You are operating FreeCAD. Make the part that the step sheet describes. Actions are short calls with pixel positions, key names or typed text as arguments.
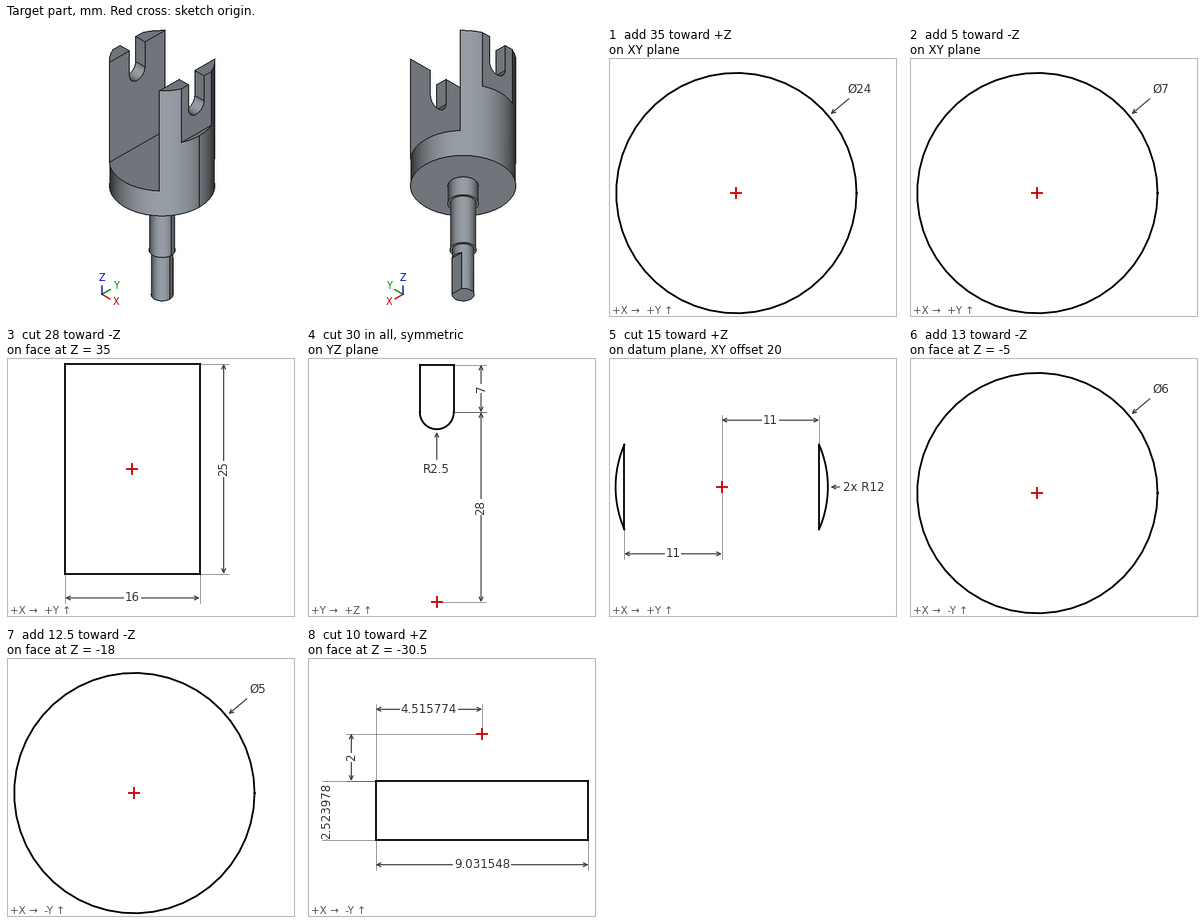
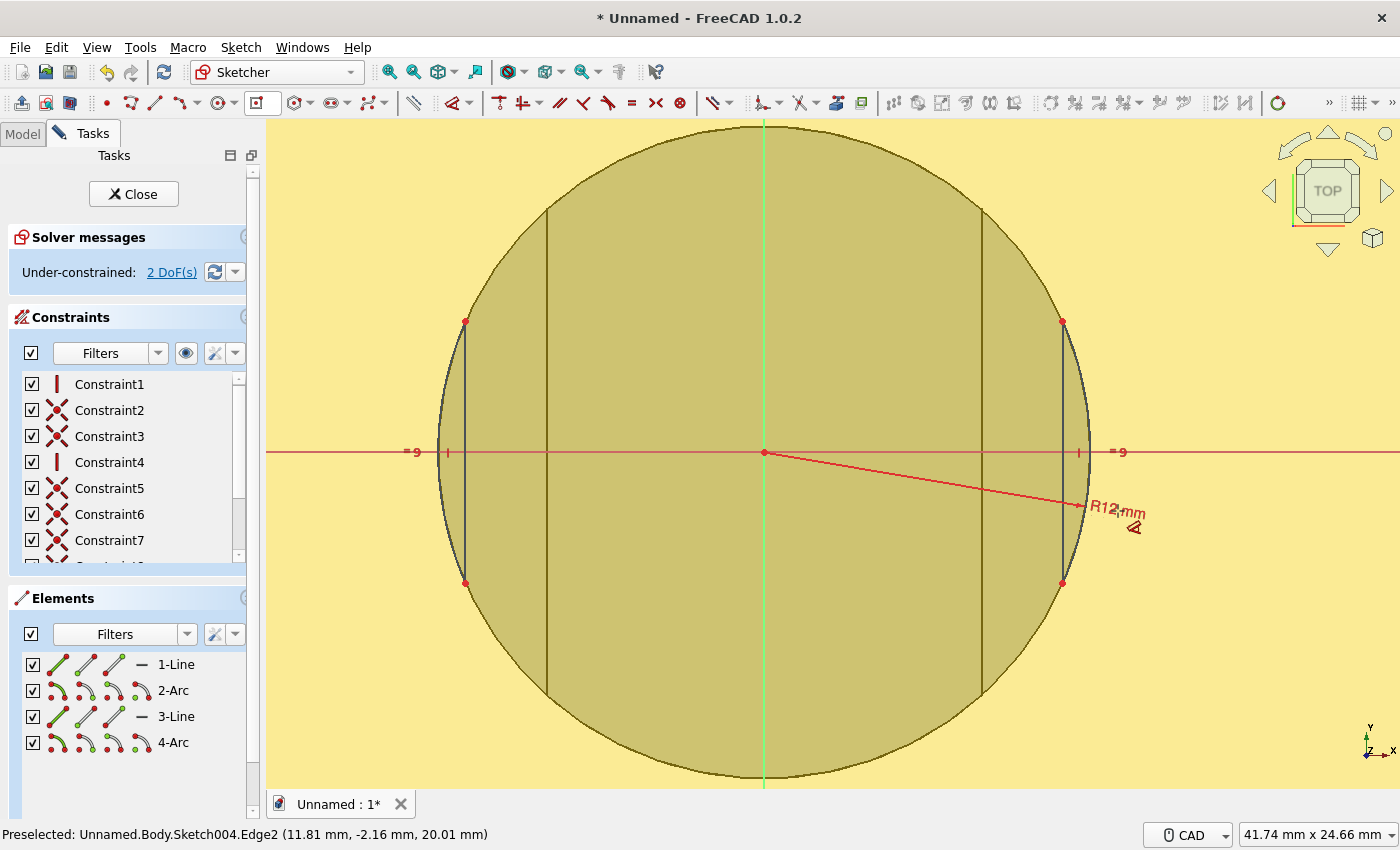
click(1063, 322)
click(914, 288)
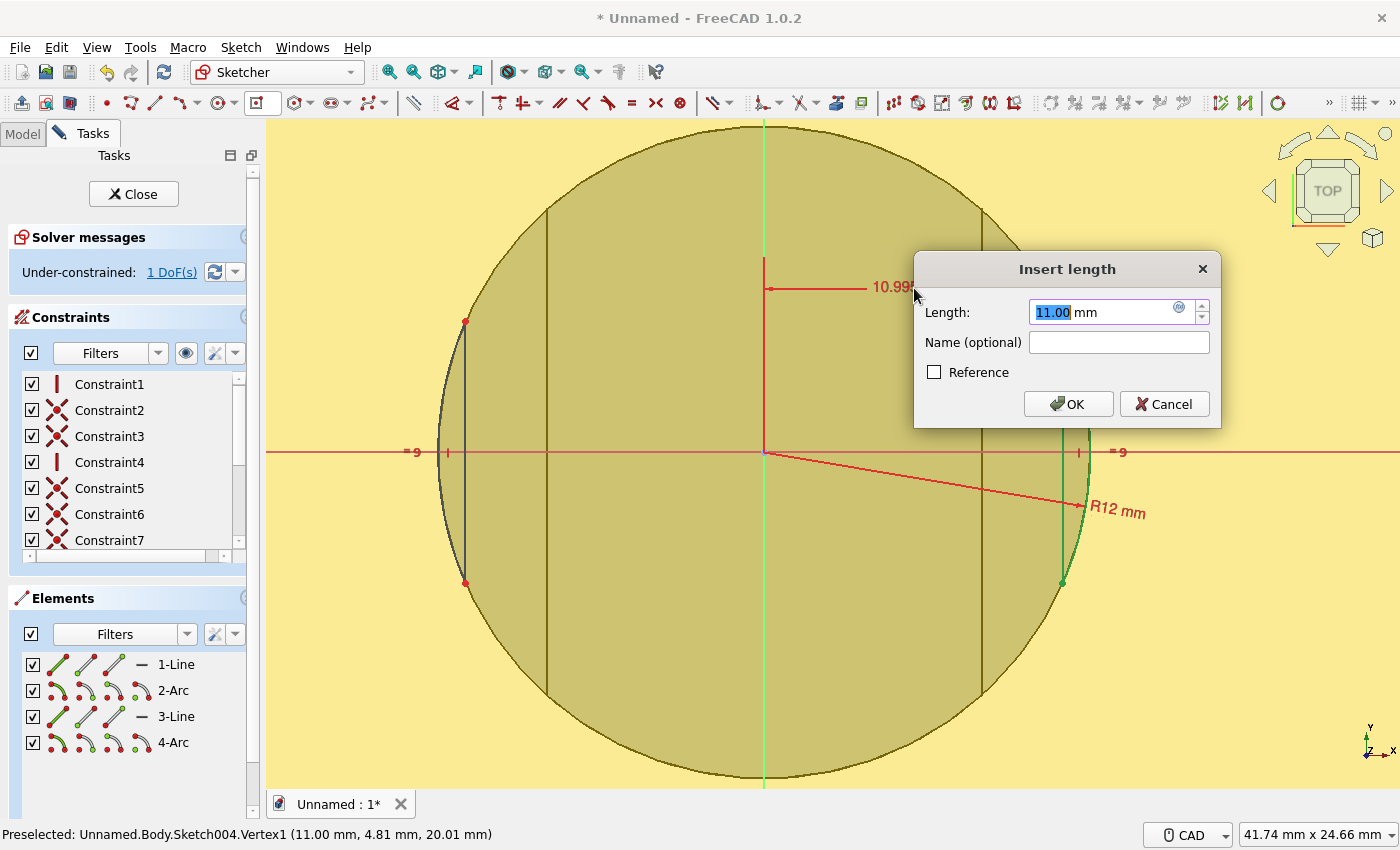
text(11)
key(Return)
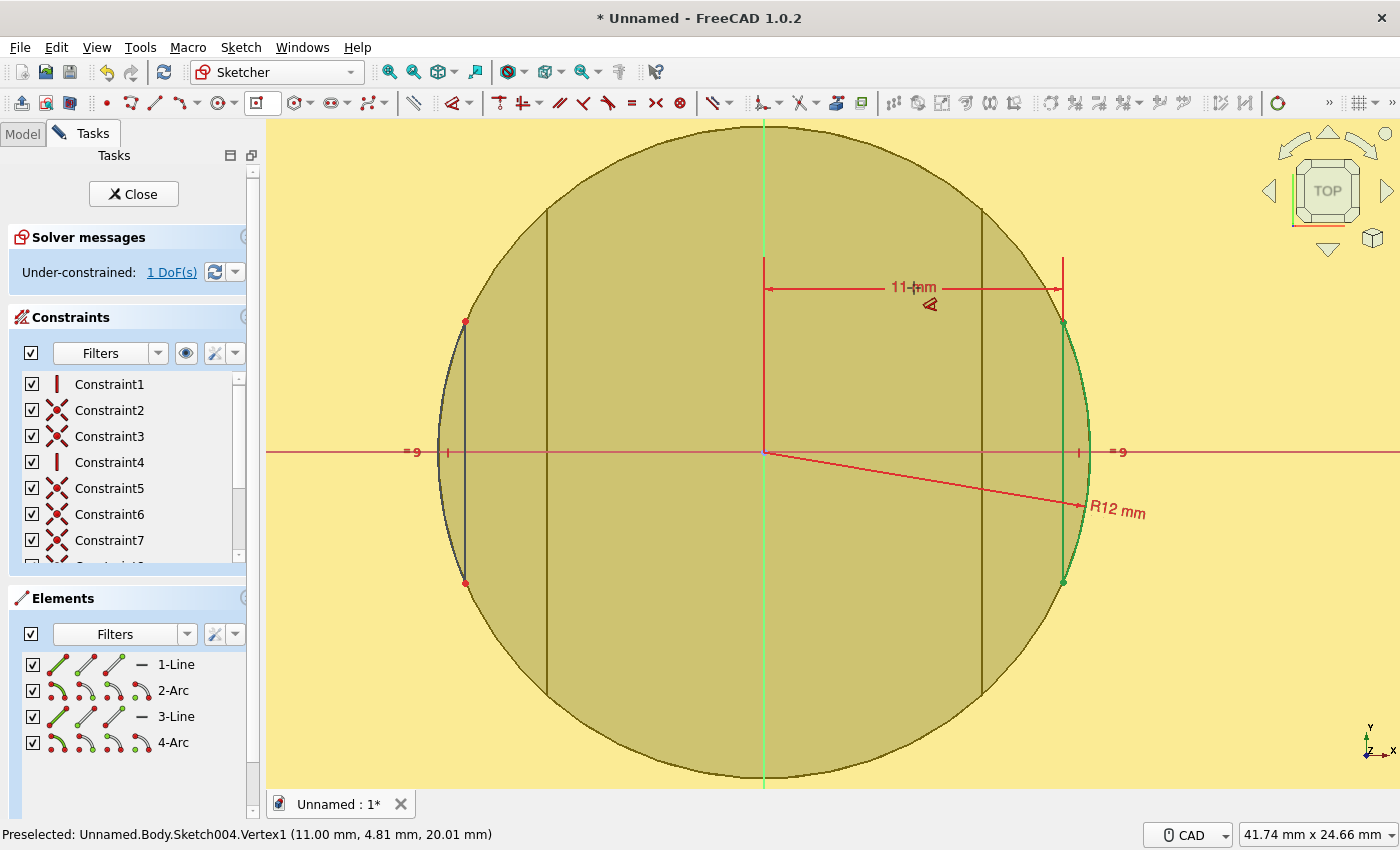
click(465, 583)
click(615, 617)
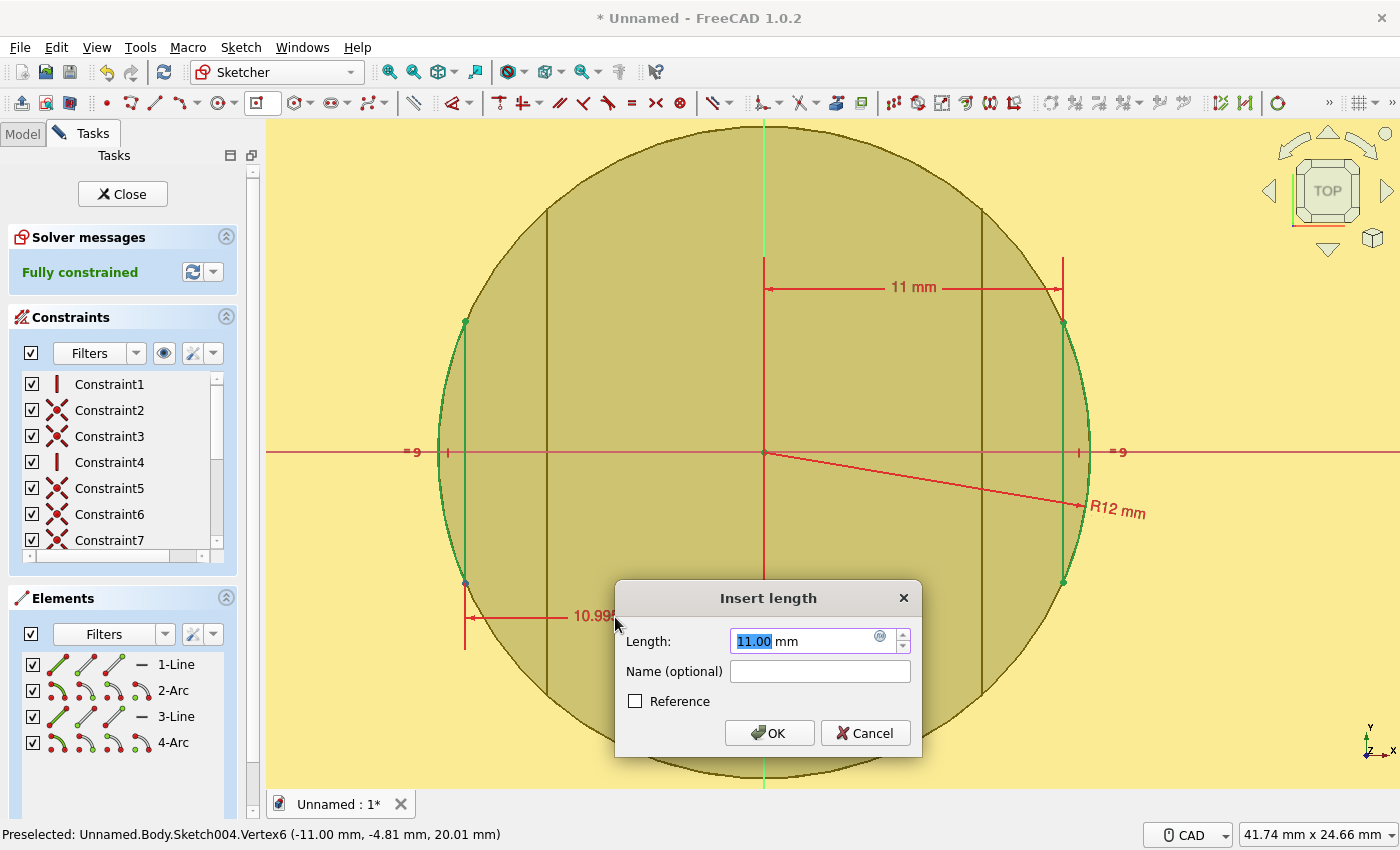
text(11)
key(Return)
key(Escape)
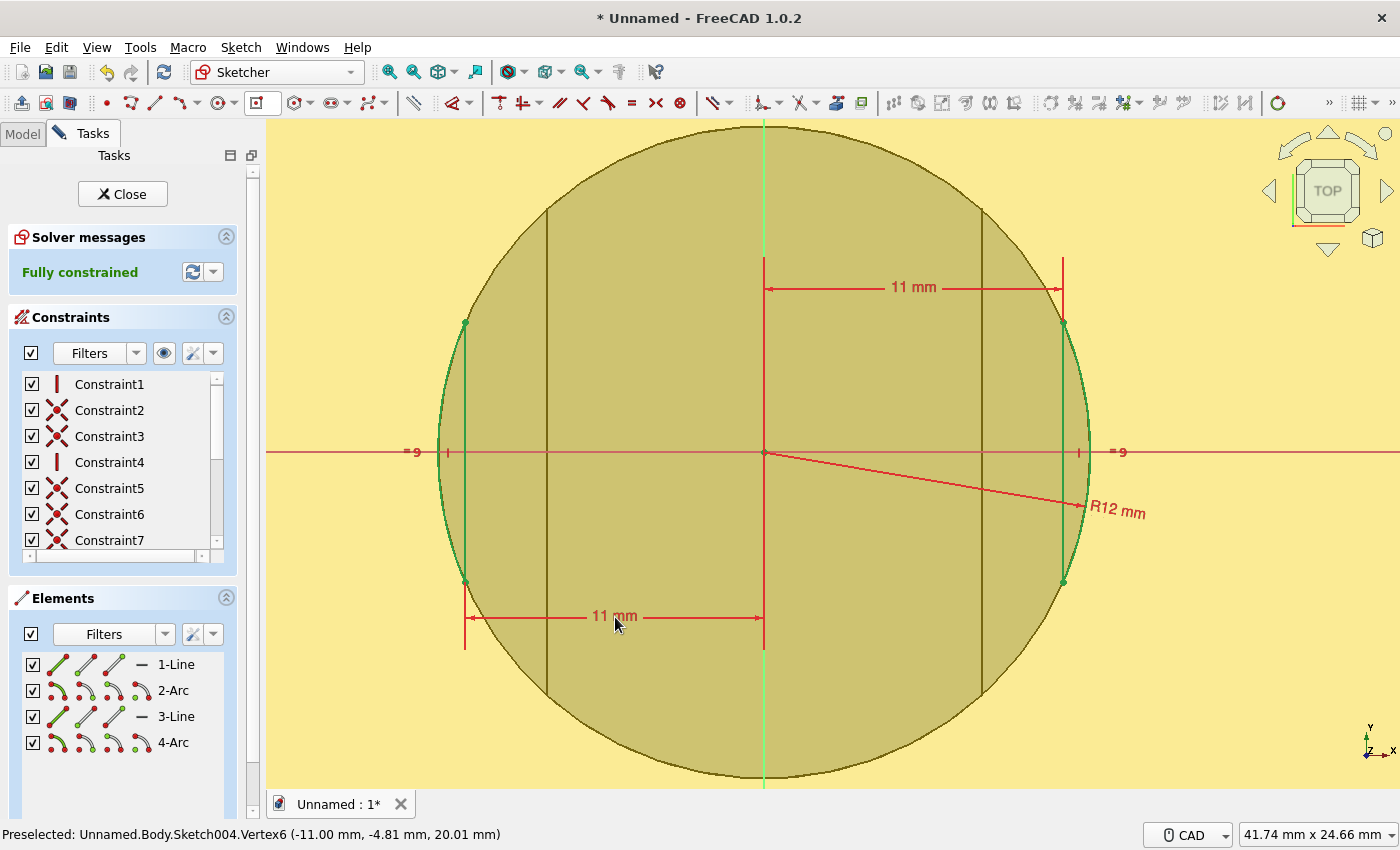
click(123, 194)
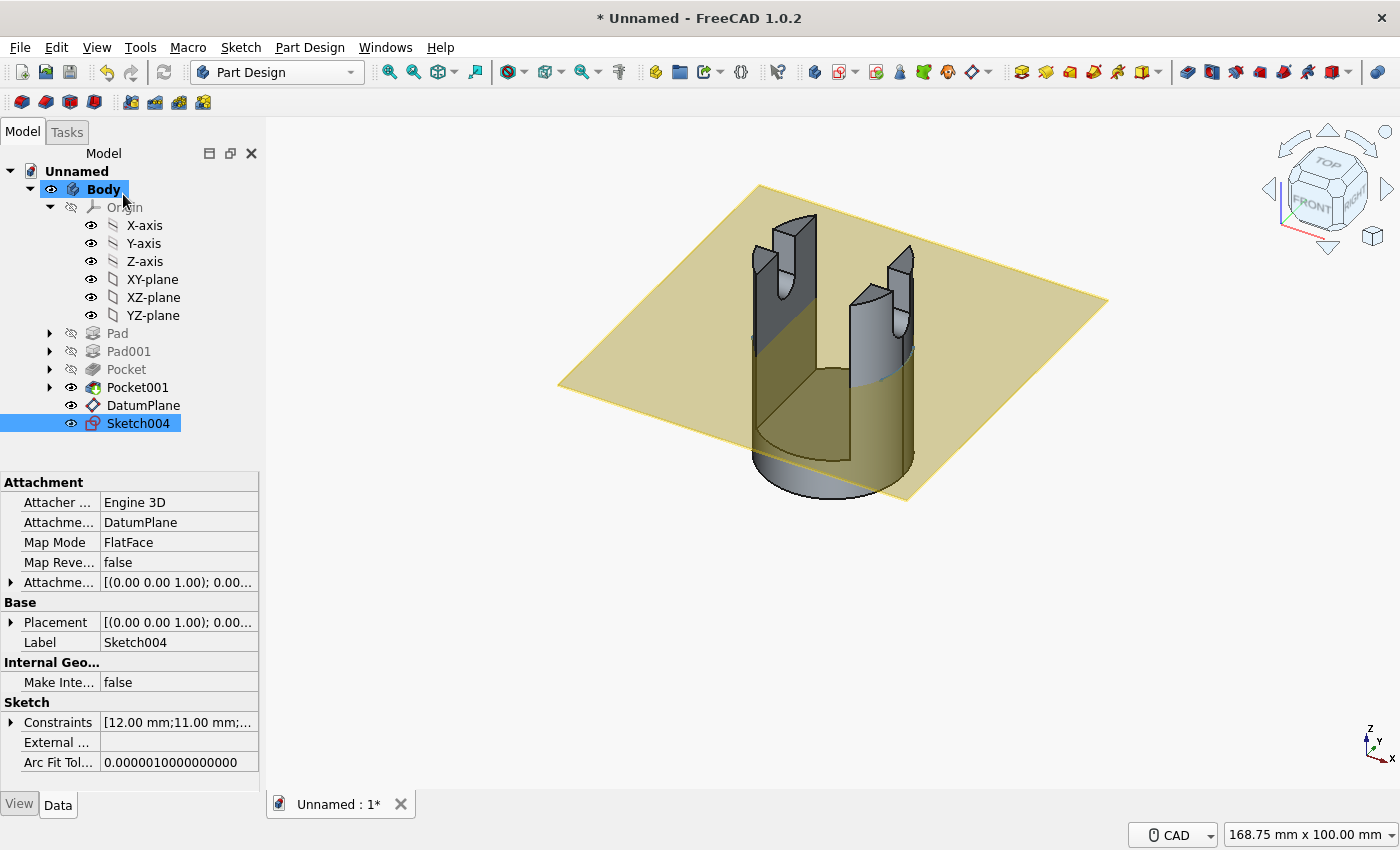
click(1188, 72)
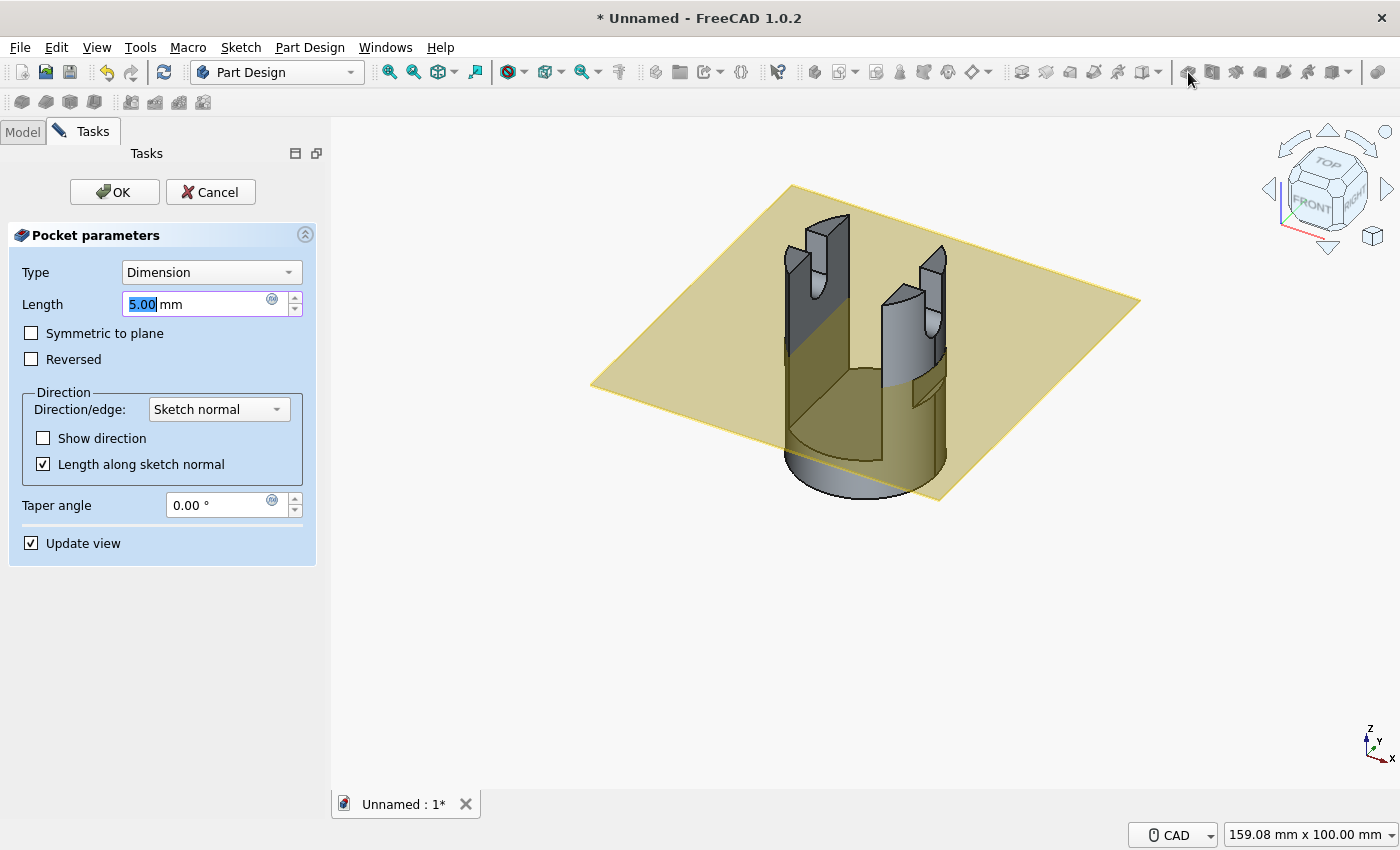
text(15)
key(Tab)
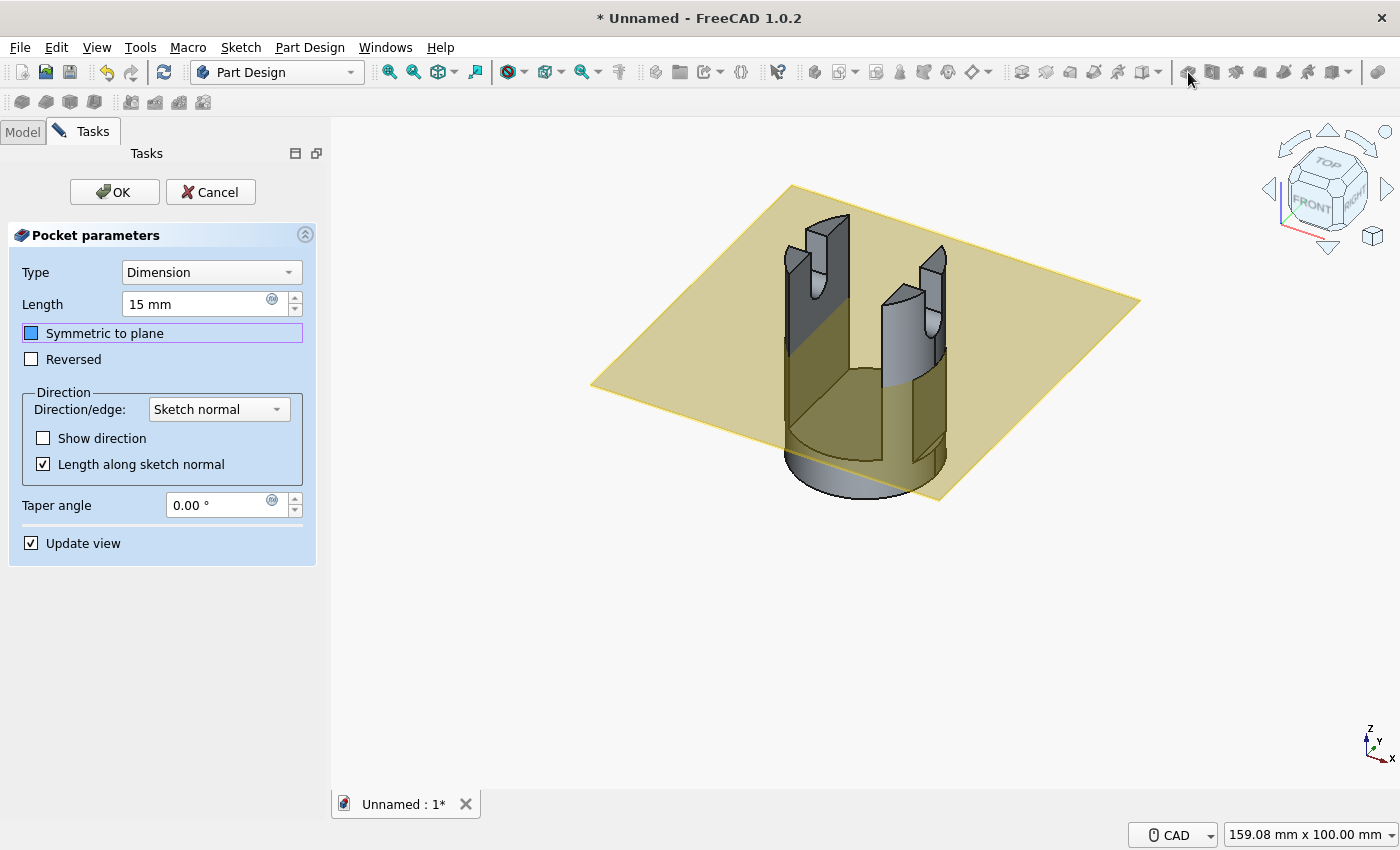
click(30, 359)